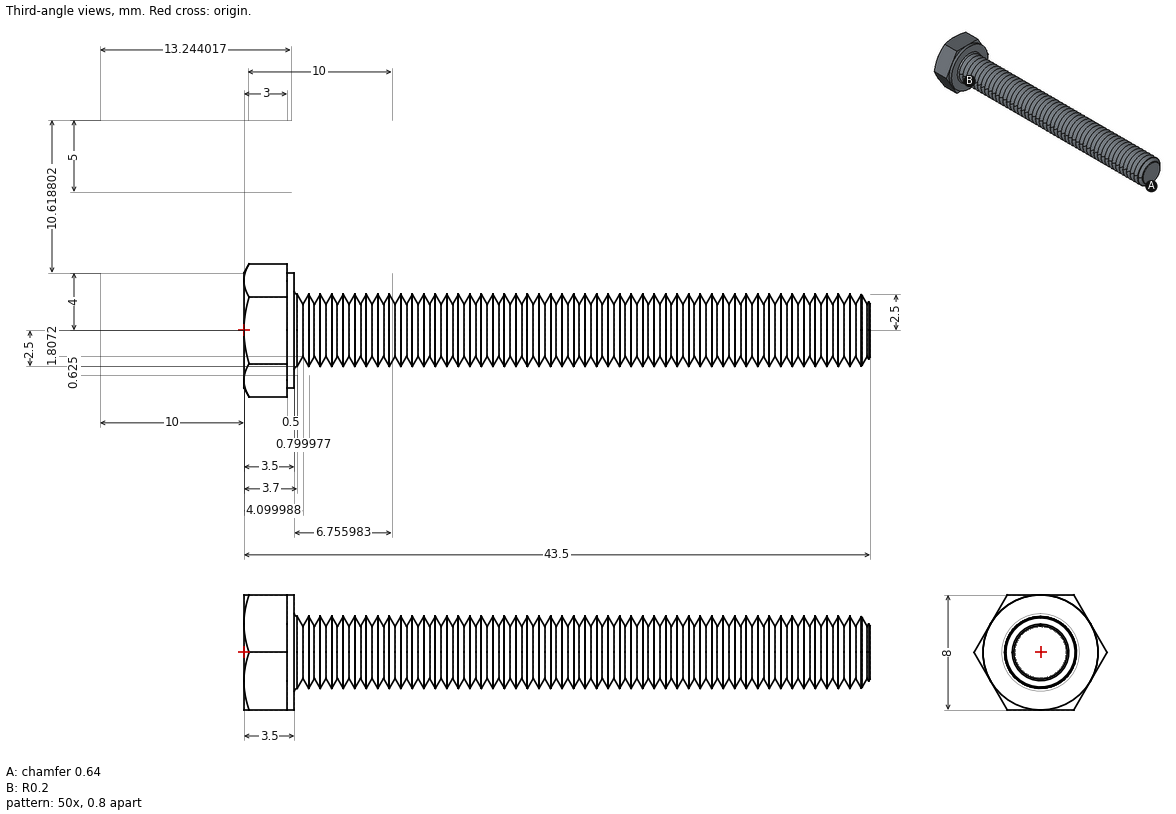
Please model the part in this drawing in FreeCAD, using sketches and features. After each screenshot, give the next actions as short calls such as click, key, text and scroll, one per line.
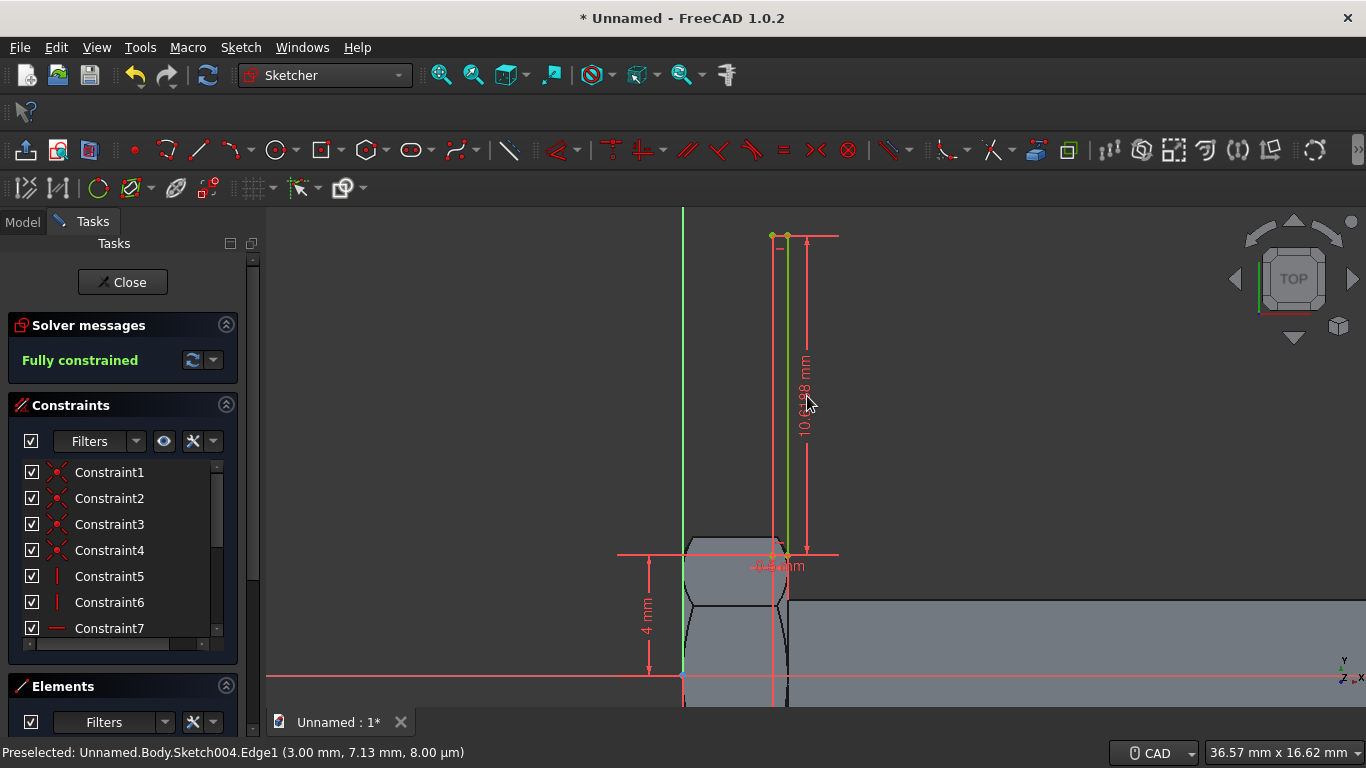
click(123, 282)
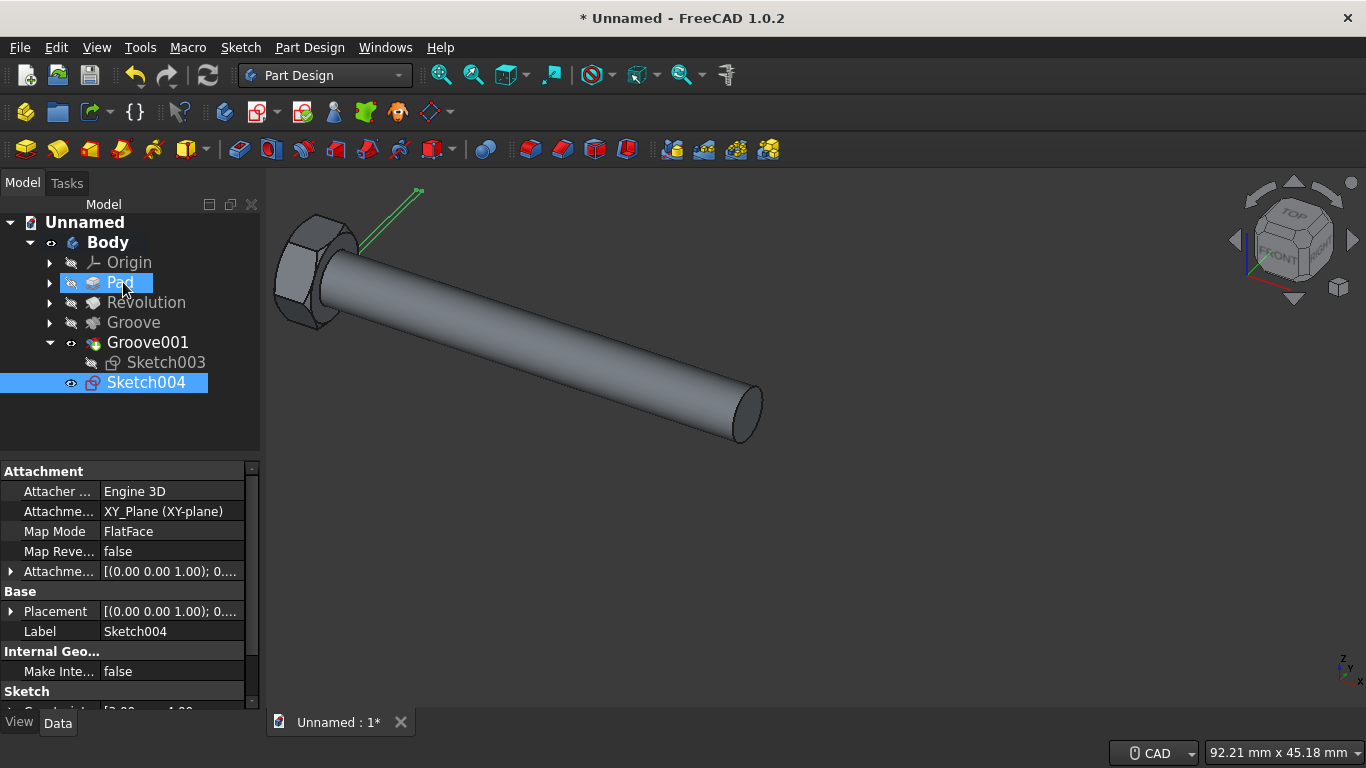
click(304, 150)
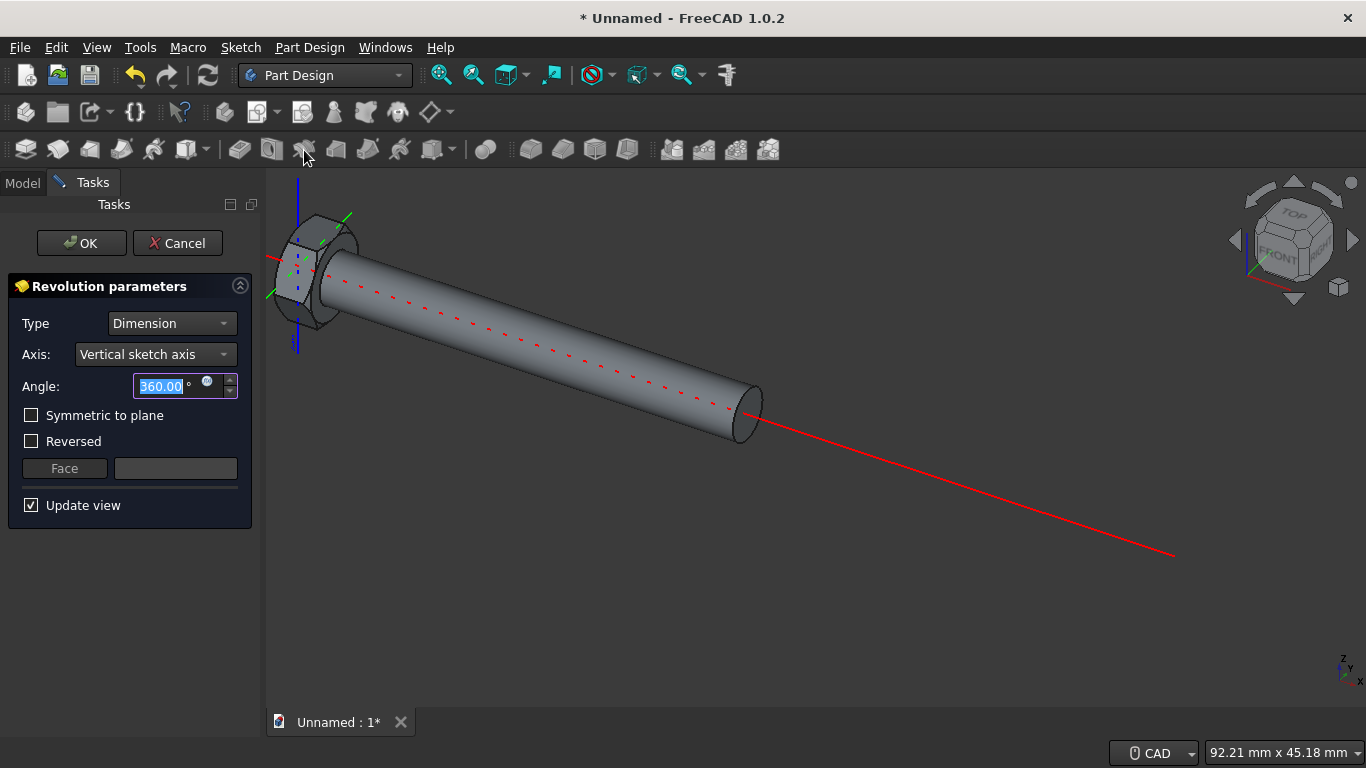
click(156, 354)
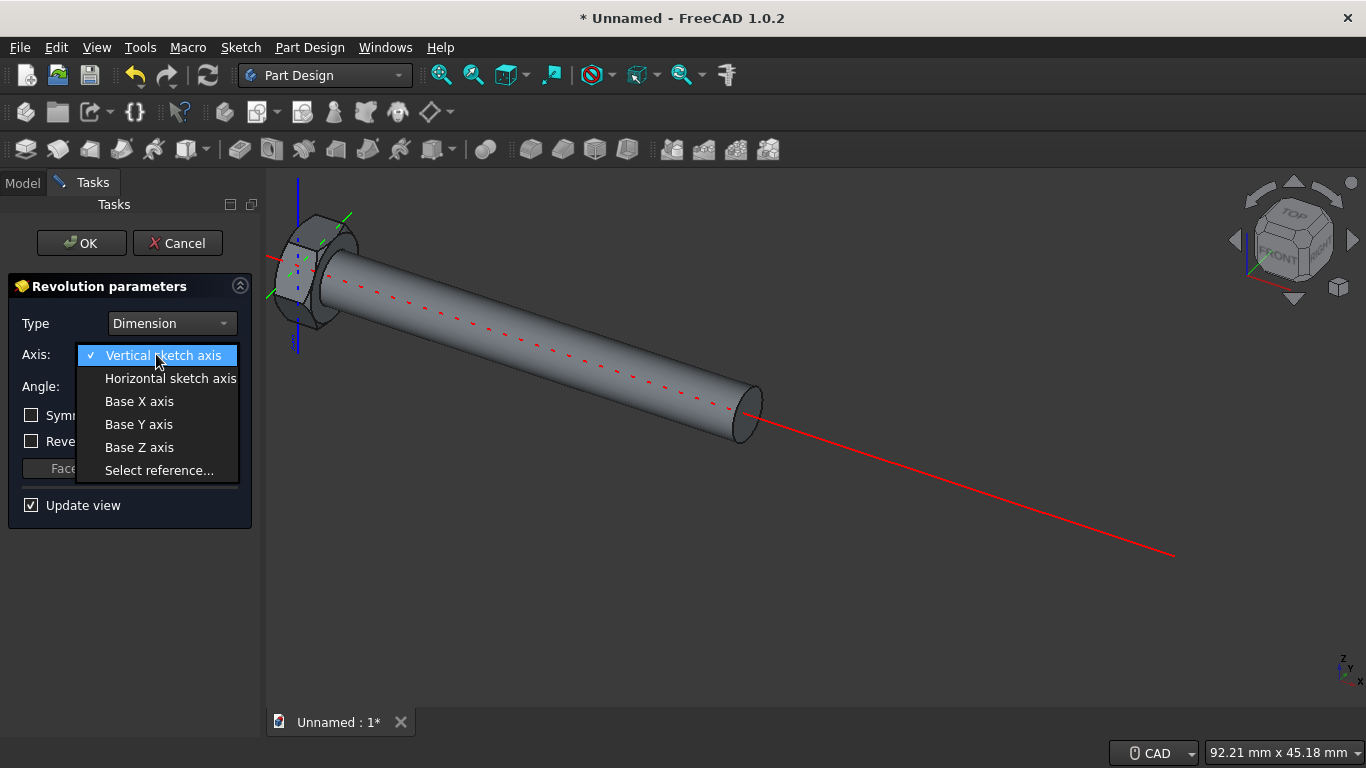
click(156, 378)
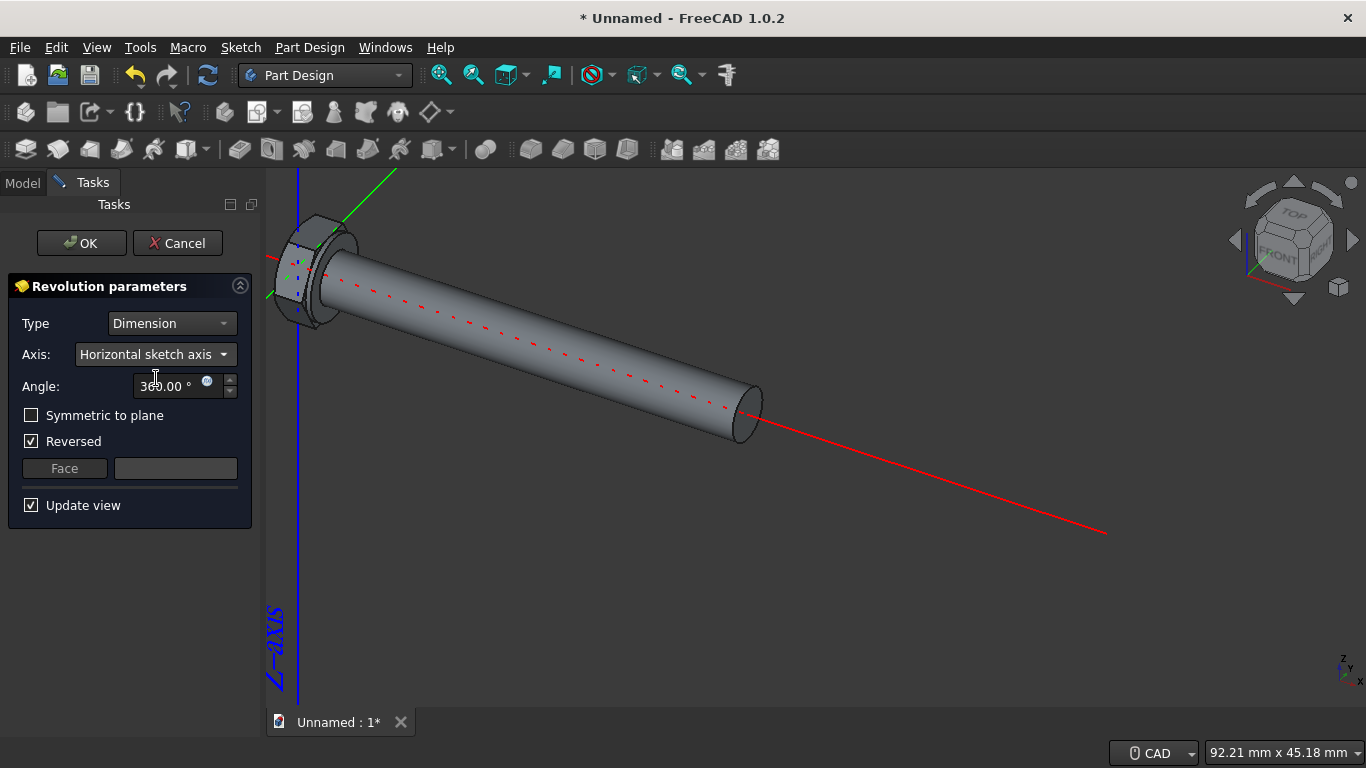
click(82, 243)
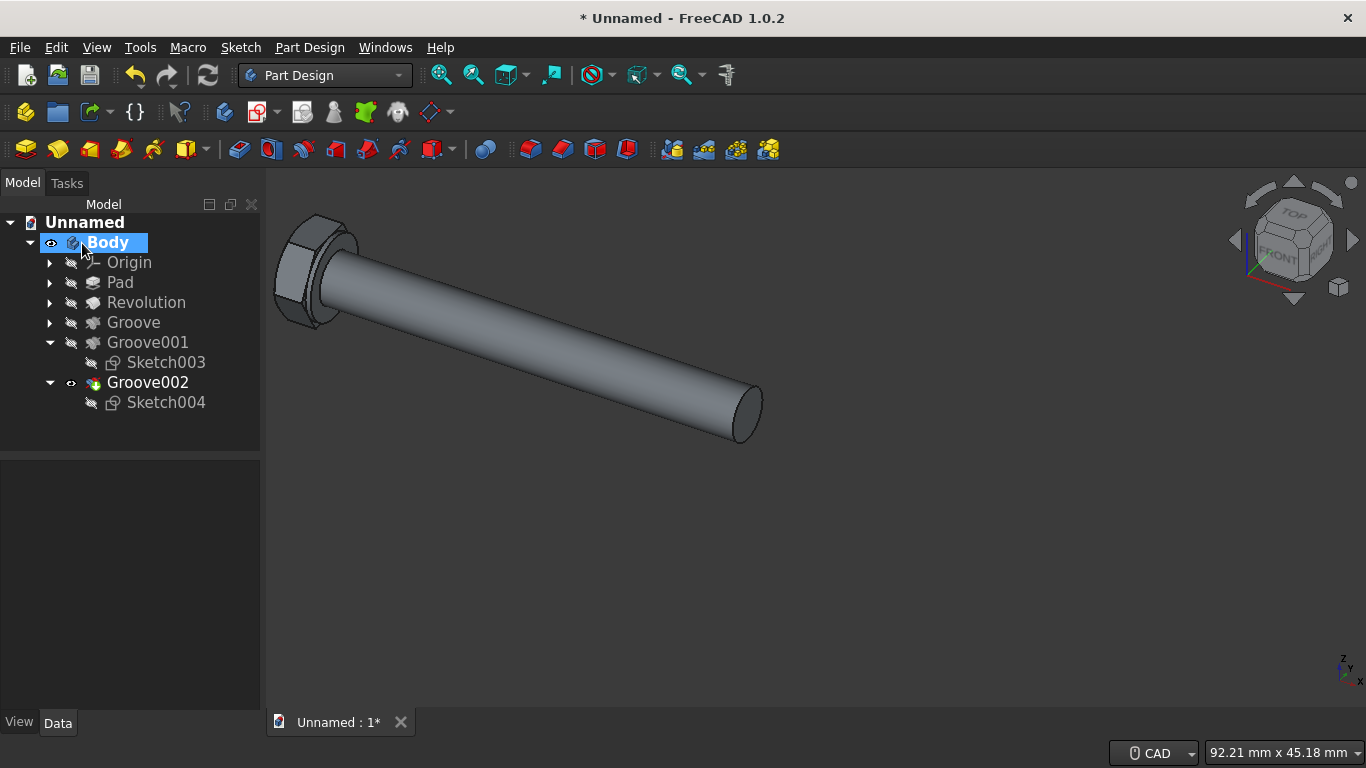
click(733, 429)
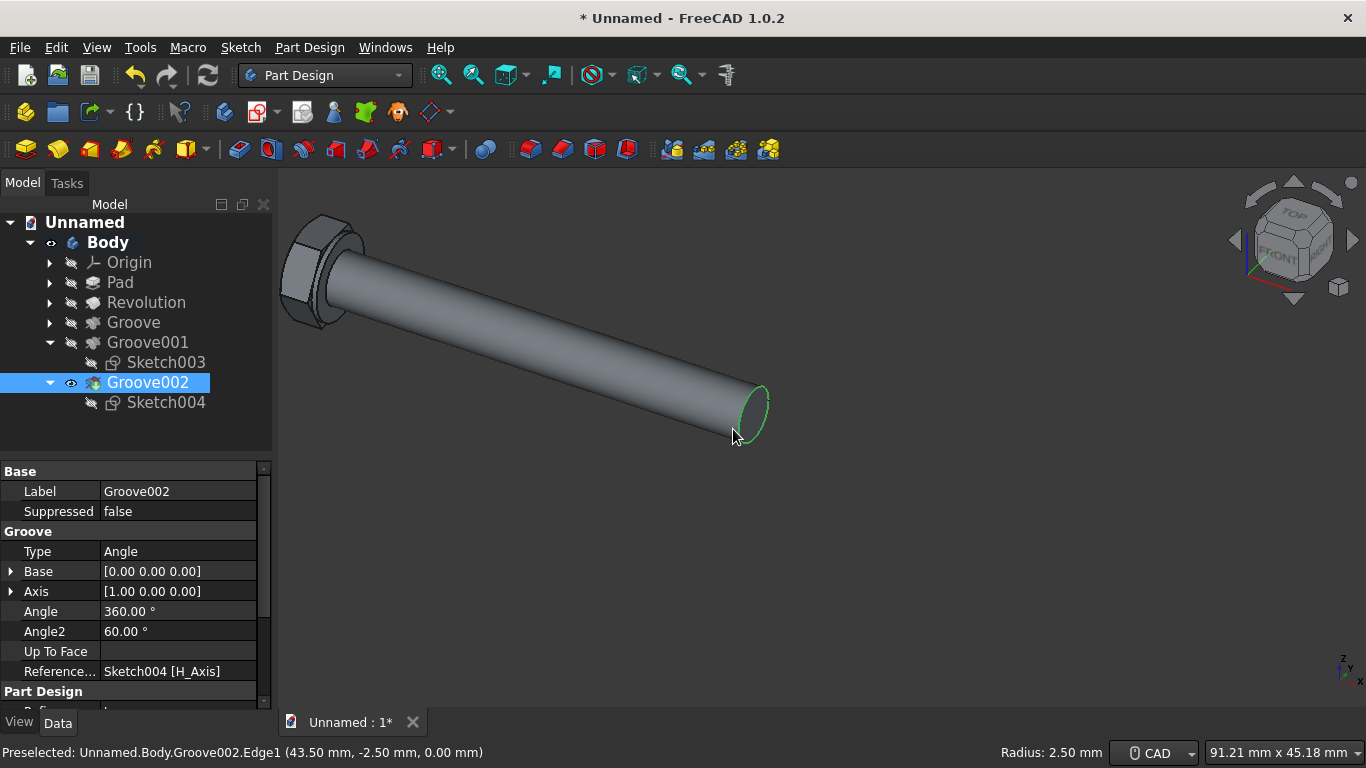
click(564, 150)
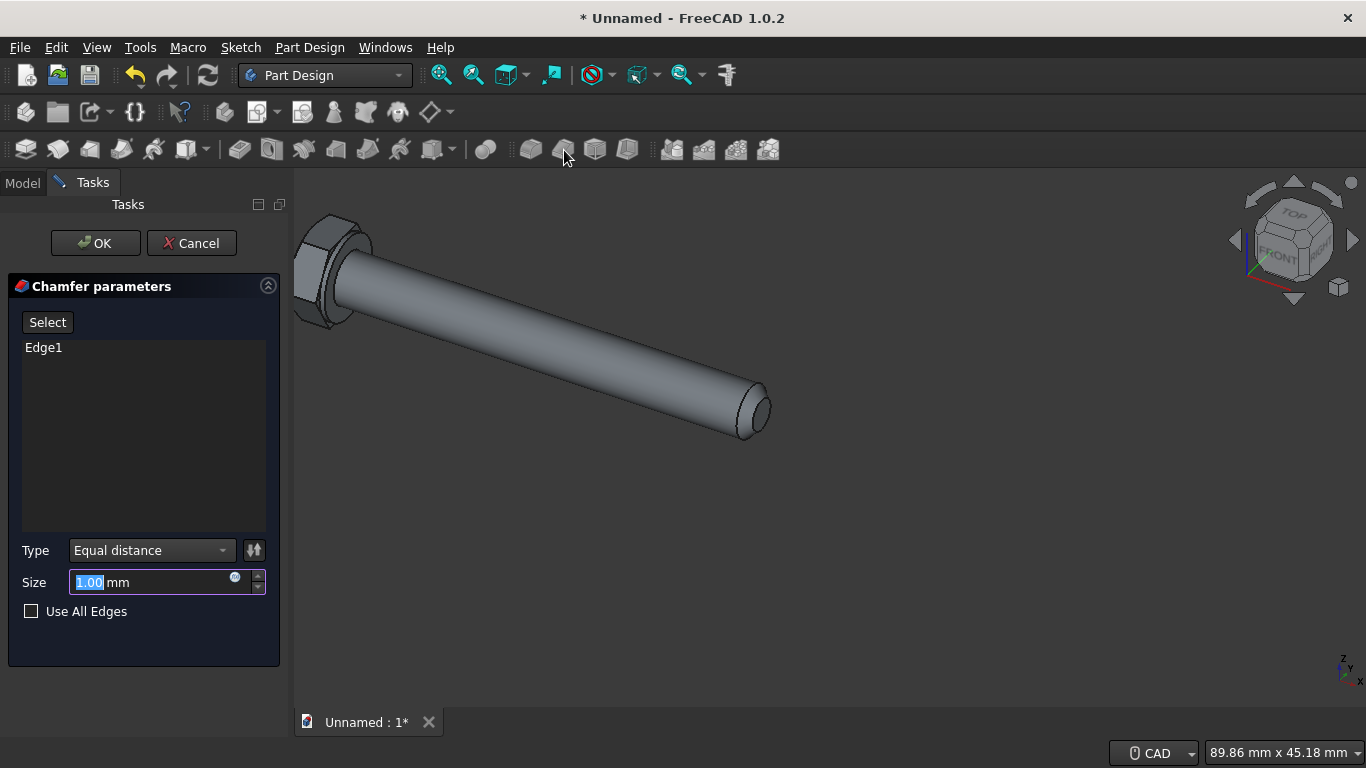
text(0.64)
key(Tab)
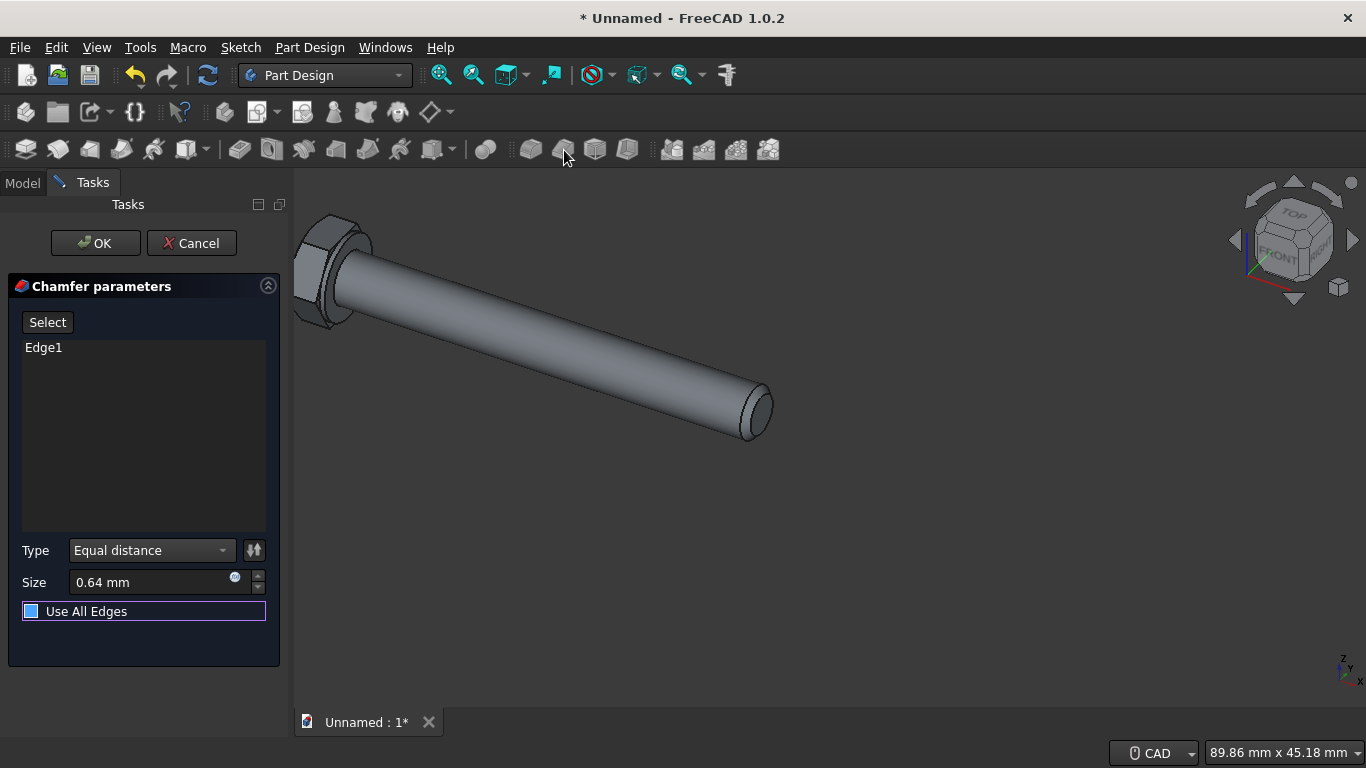
click(96, 243)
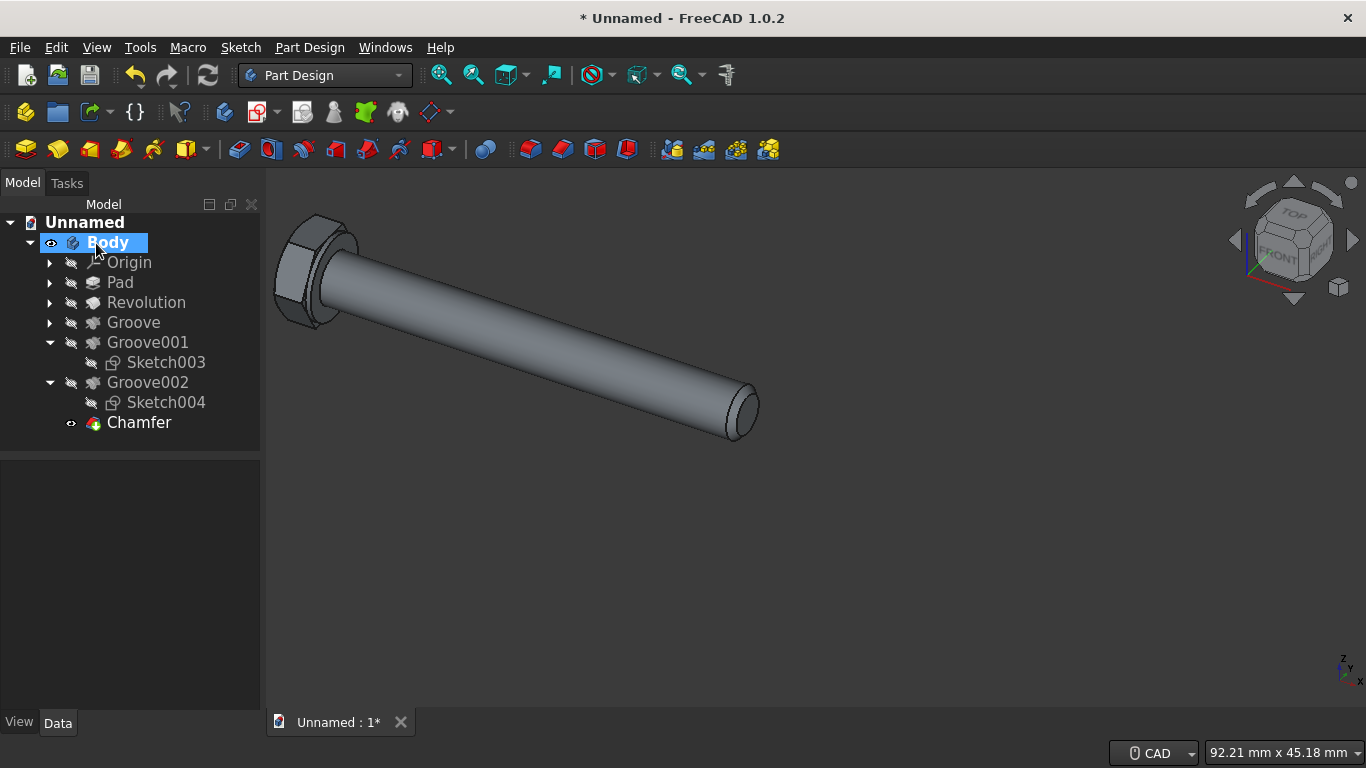
key(0)